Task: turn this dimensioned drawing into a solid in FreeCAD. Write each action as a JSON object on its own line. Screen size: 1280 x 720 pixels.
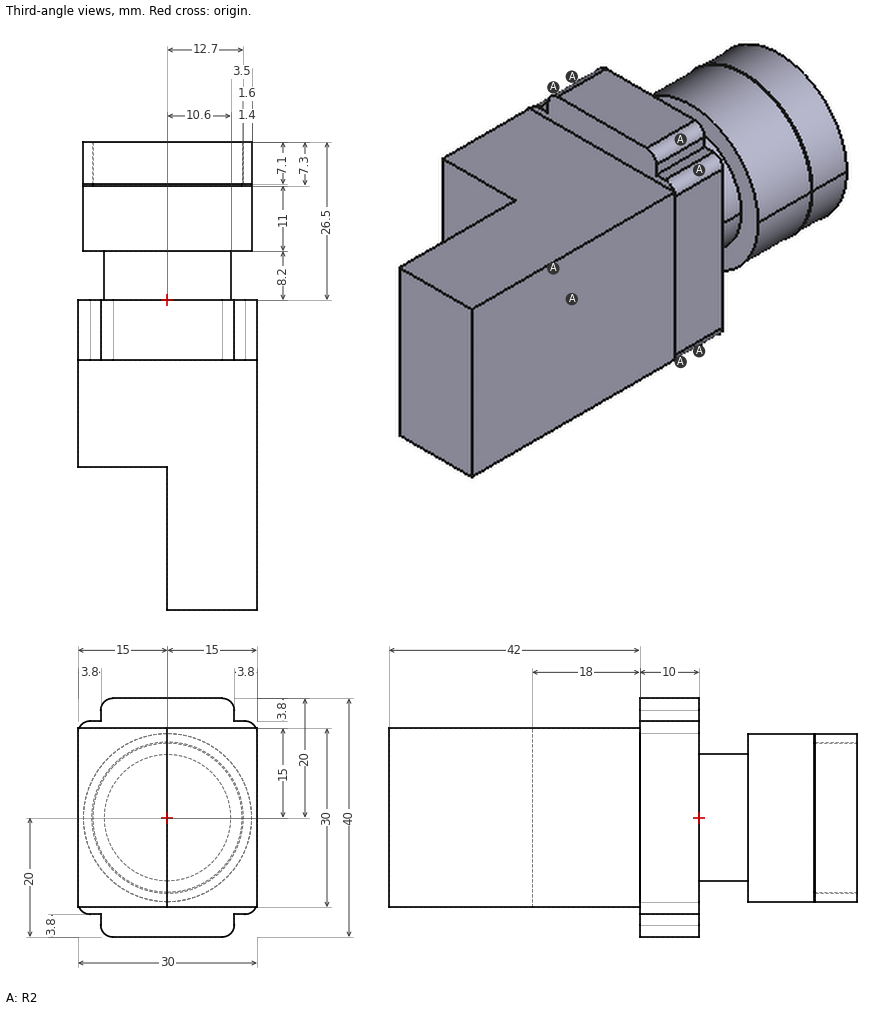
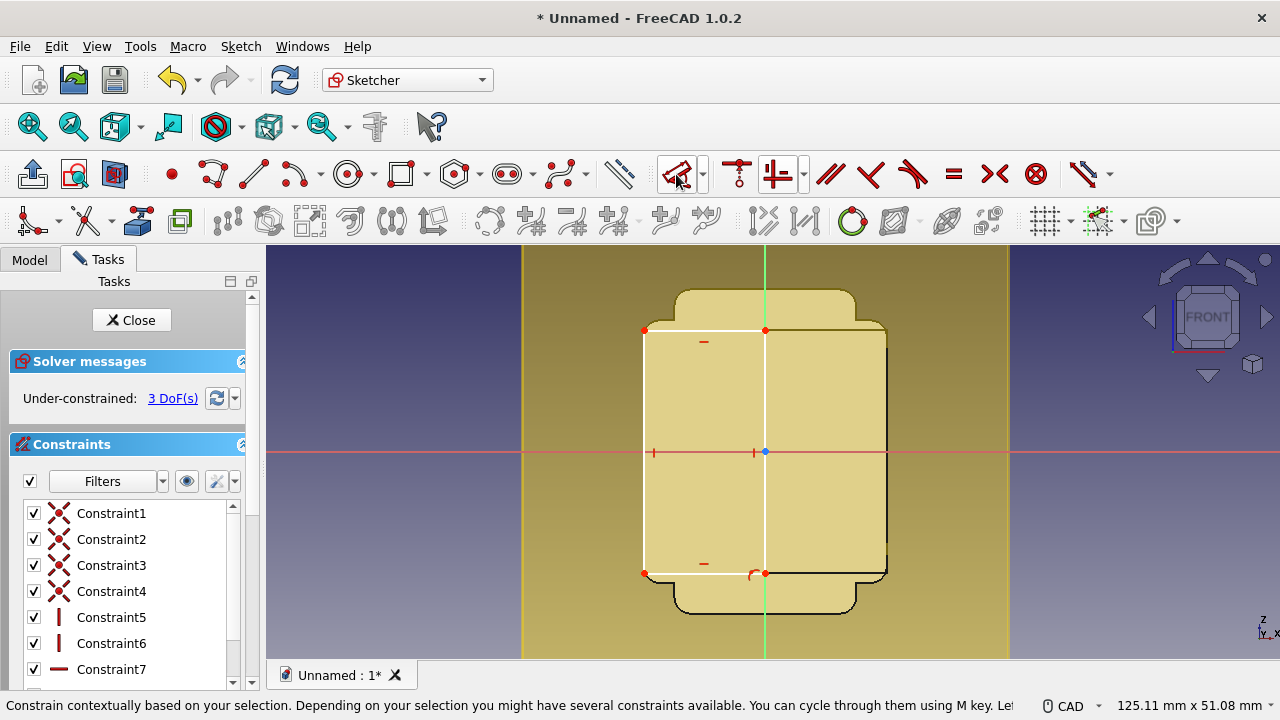
{"action": "left_click", "coordinate": [644, 404]}
{"action": "left_click", "coordinate": [610, 397]}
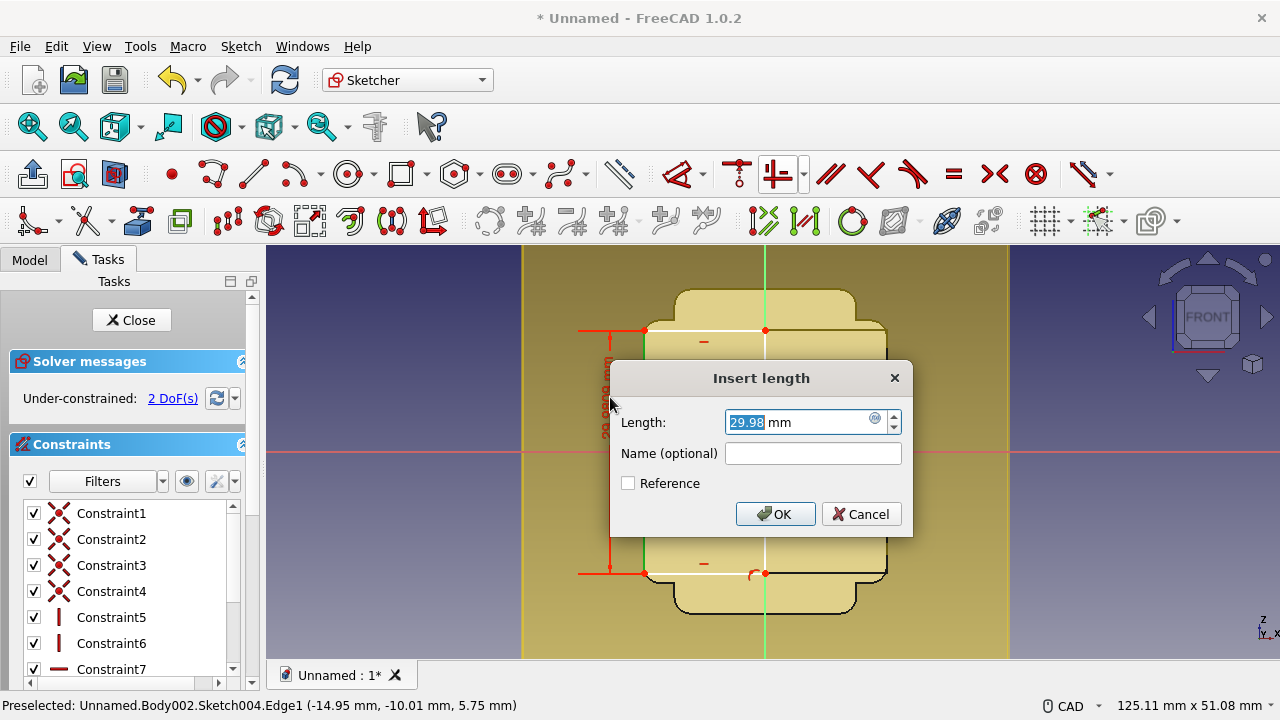
{"action": "type", "text": "30"}
{"action": "key", "text": "Return"}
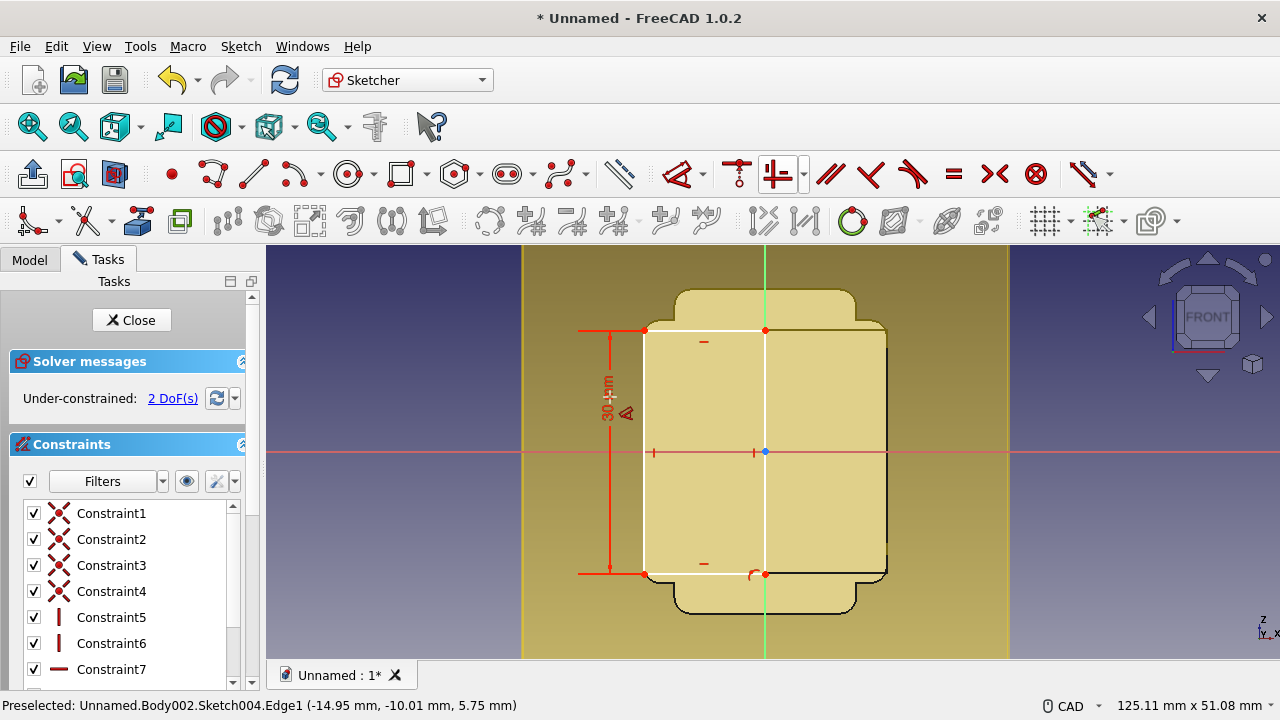
{"action": "left_click", "coordinate": [680, 574]}
{"action": "left_click", "coordinate": [705, 608]}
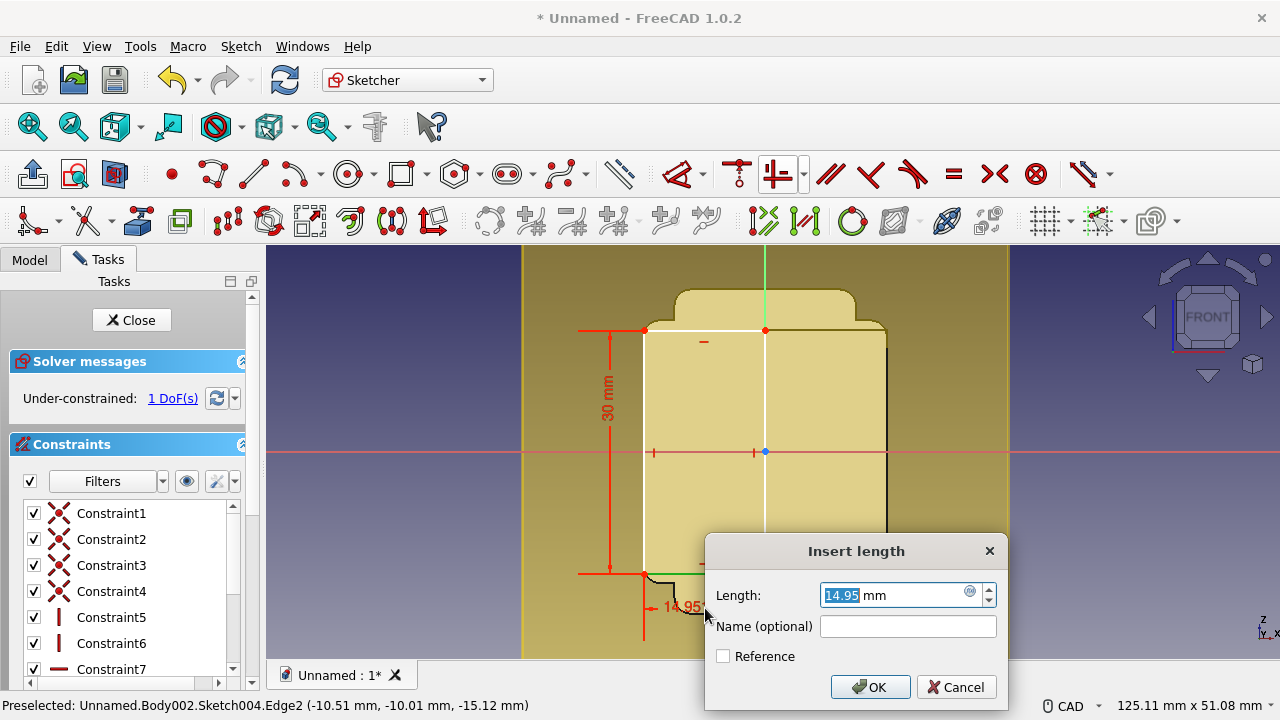
{"action": "type", "text": "15"}
{"action": "key", "text": "Return"}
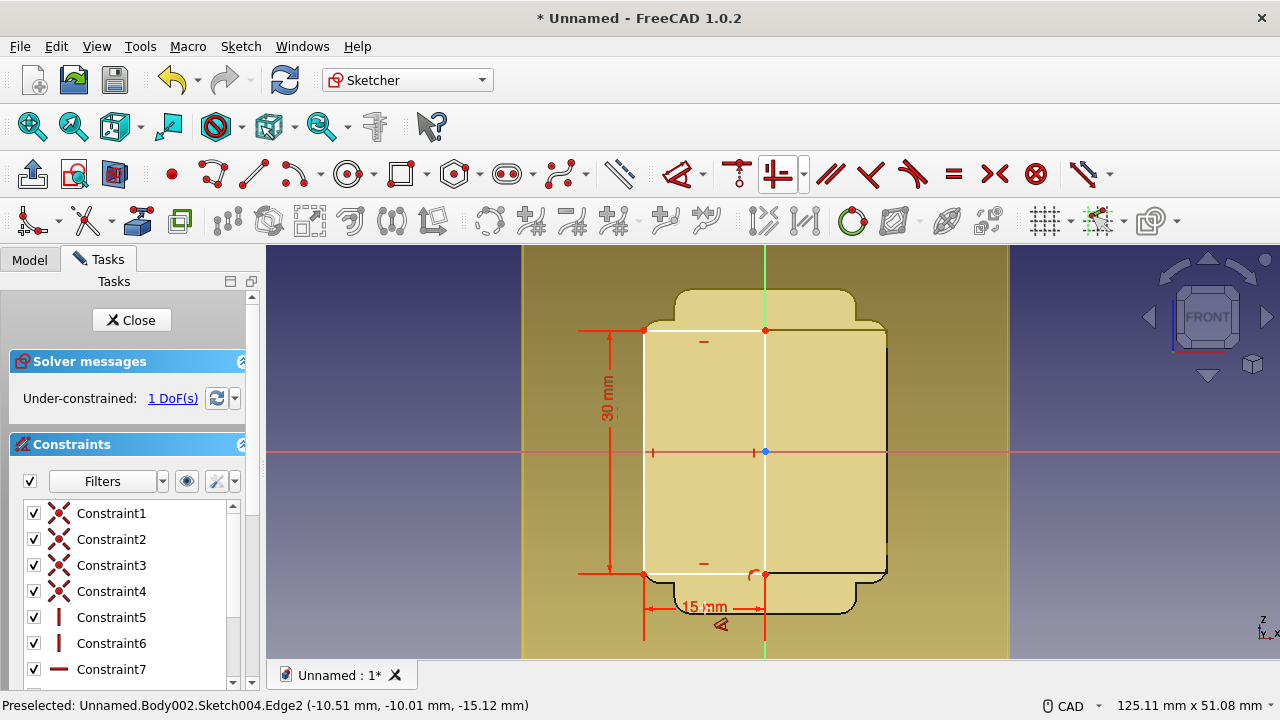
{"action": "left_click", "coordinate": [644, 331]}
{"action": "left_click", "coordinate": [799, 391]}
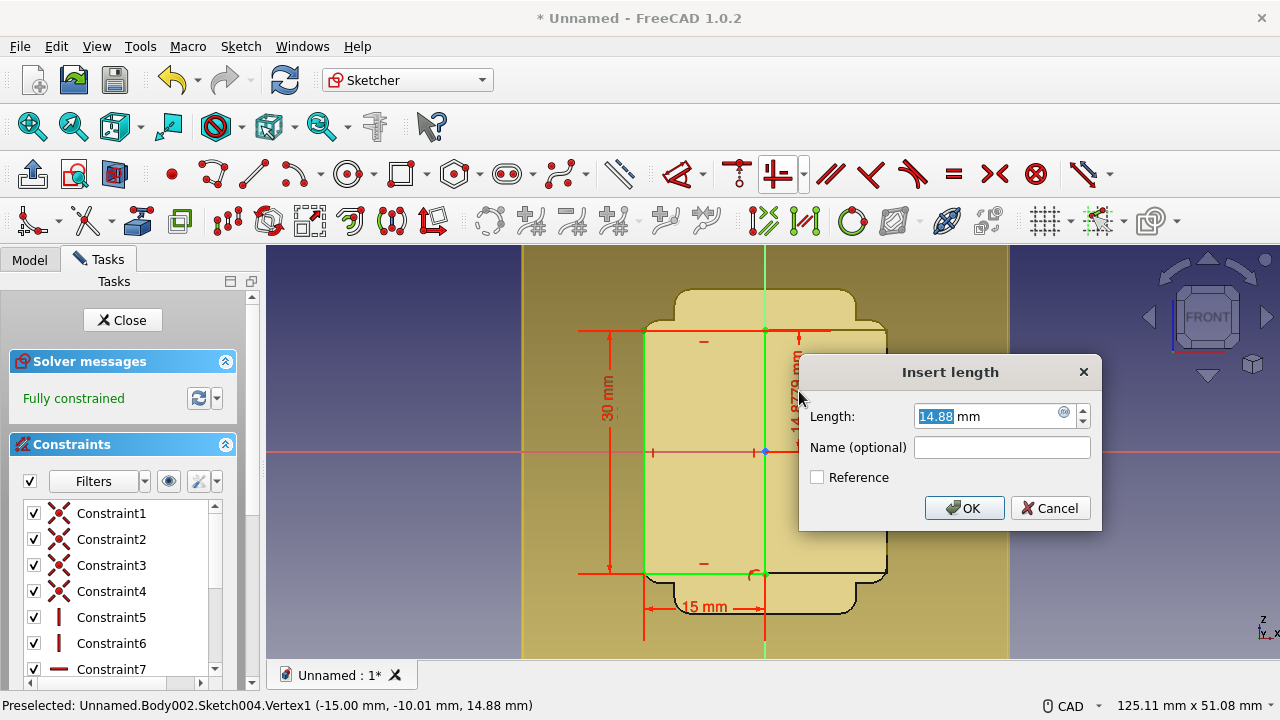
{"action": "type", "text": "15"}
{"action": "key", "text": "Return"}
{"action": "key", "text": "Escape"}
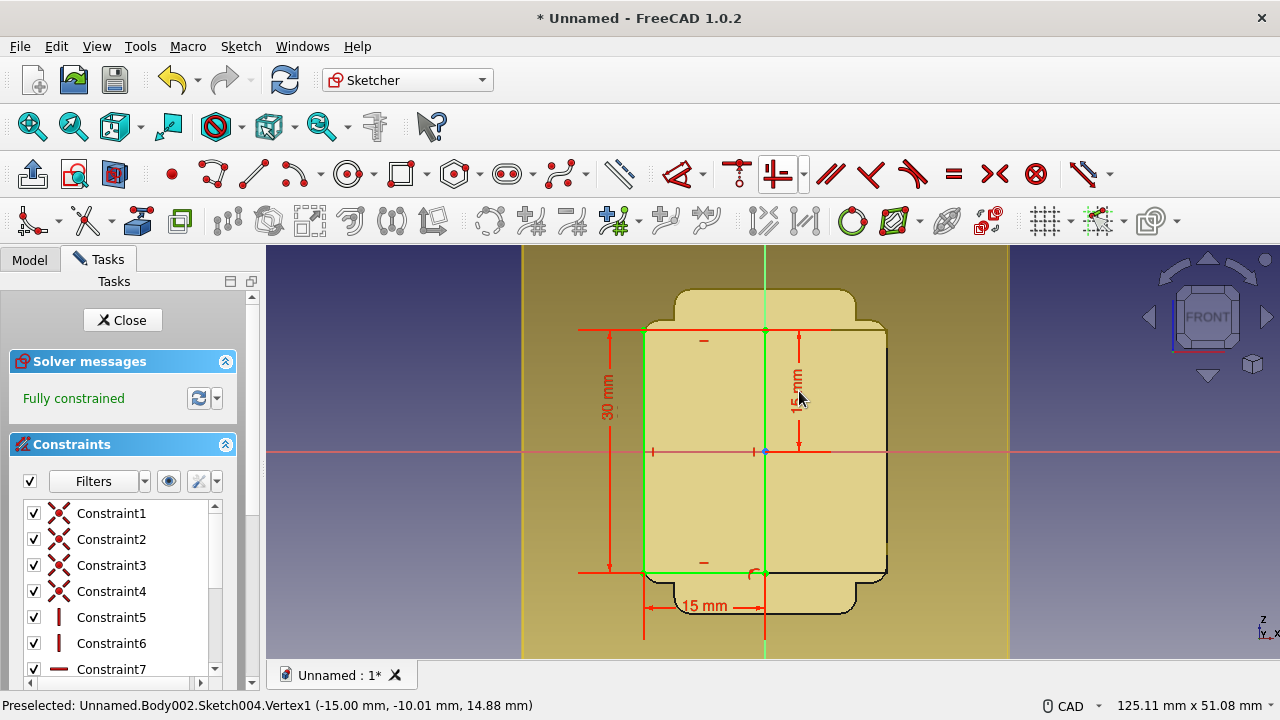
{"action": "left_click", "coordinate": [123, 320]}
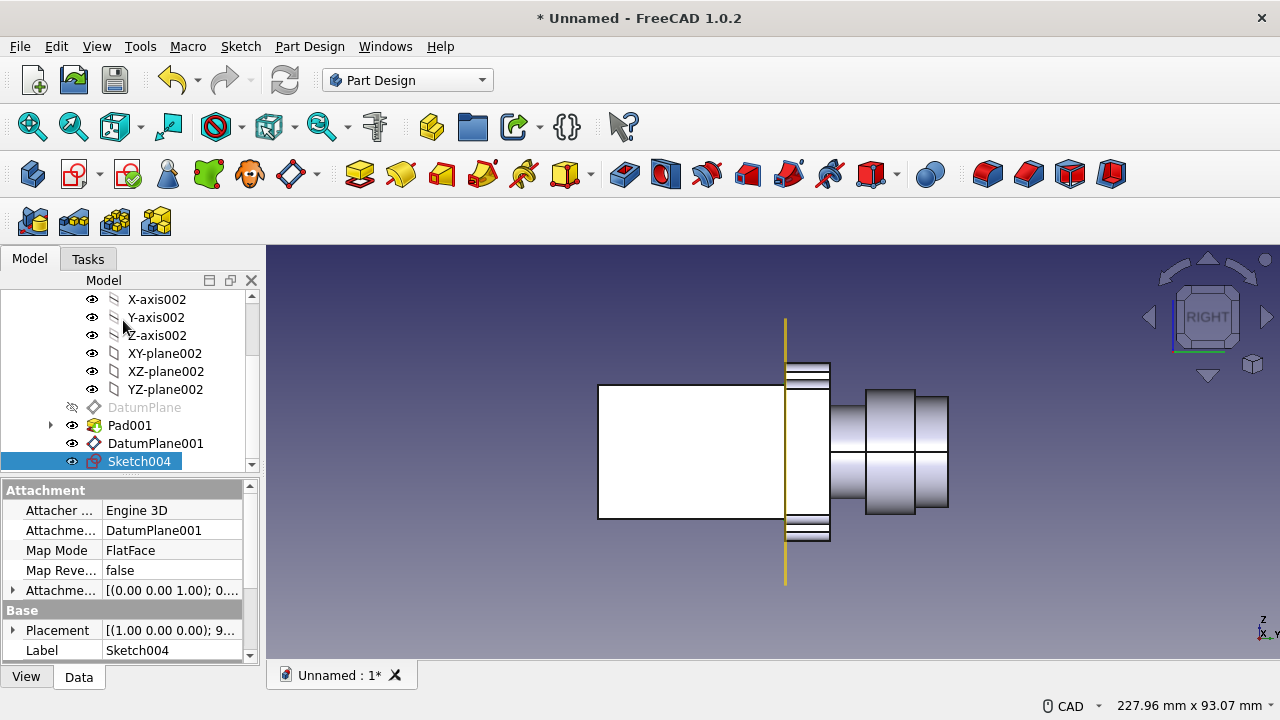
{"action": "left_click", "coordinate": [360, 174]}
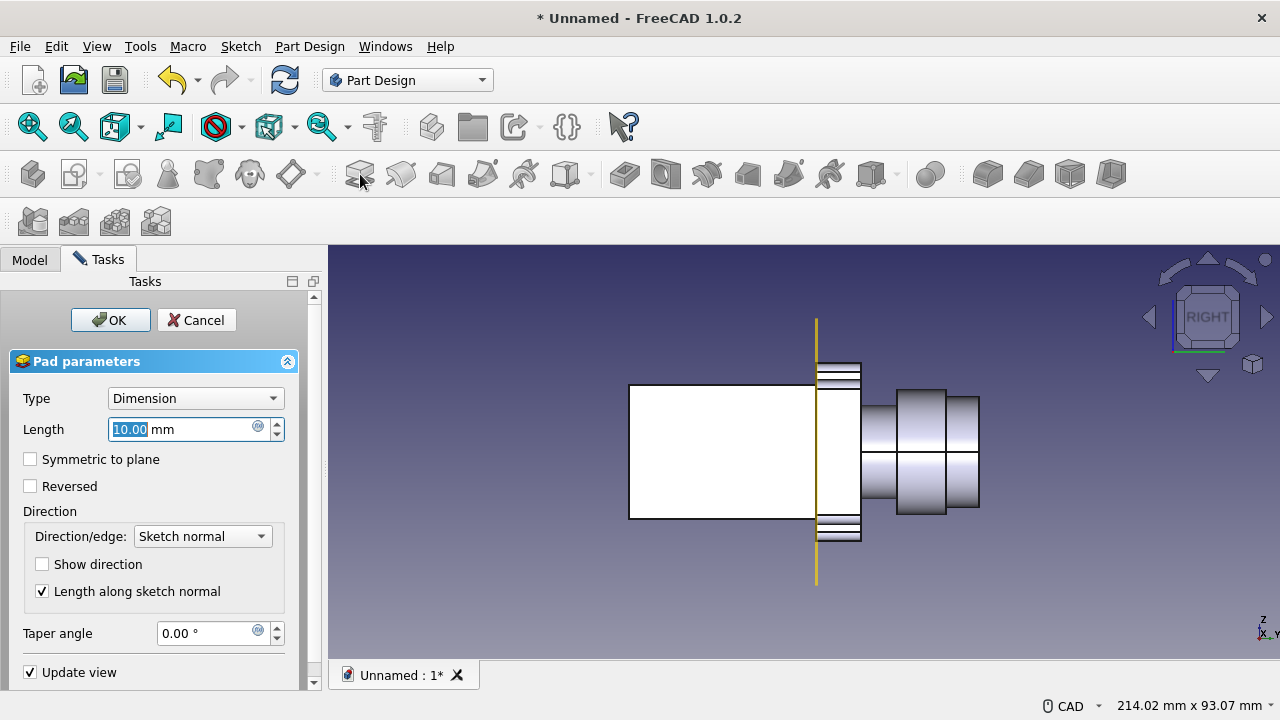
{"action": "type", "text": "18"}
{"action": "key", "text": "Tab"}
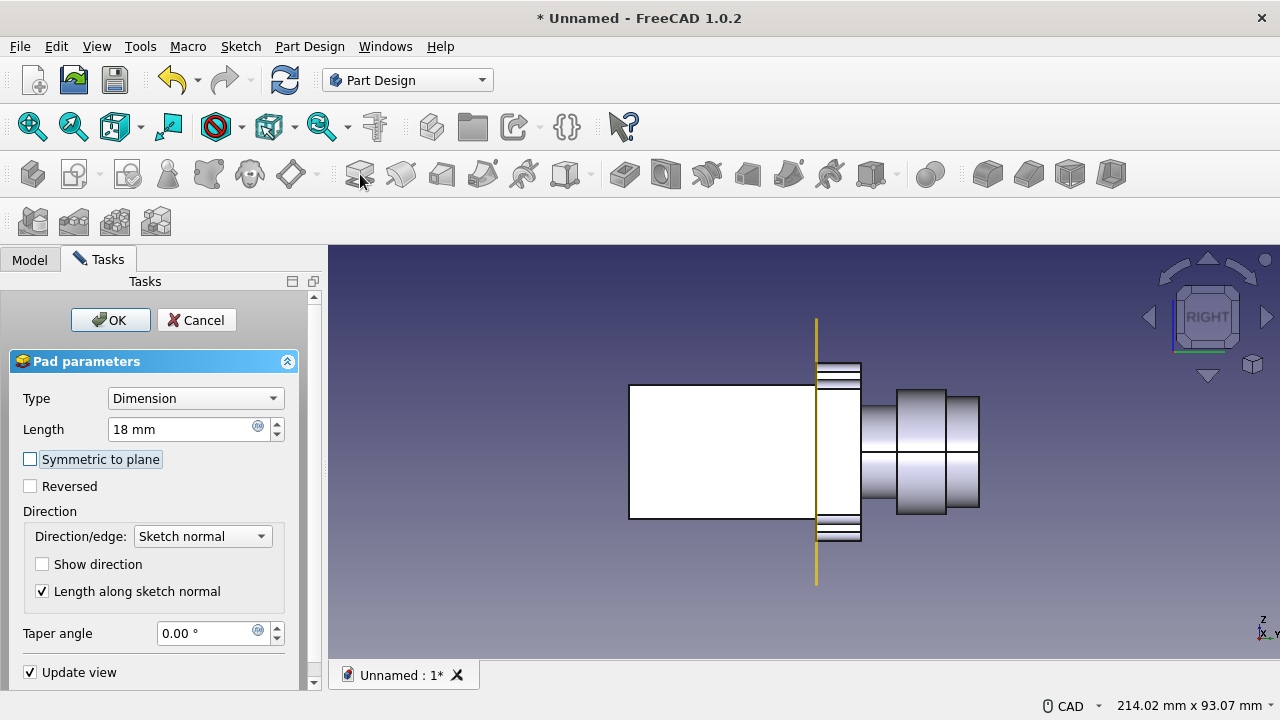
{"action": "left_click", "coordinate": [111, 320]}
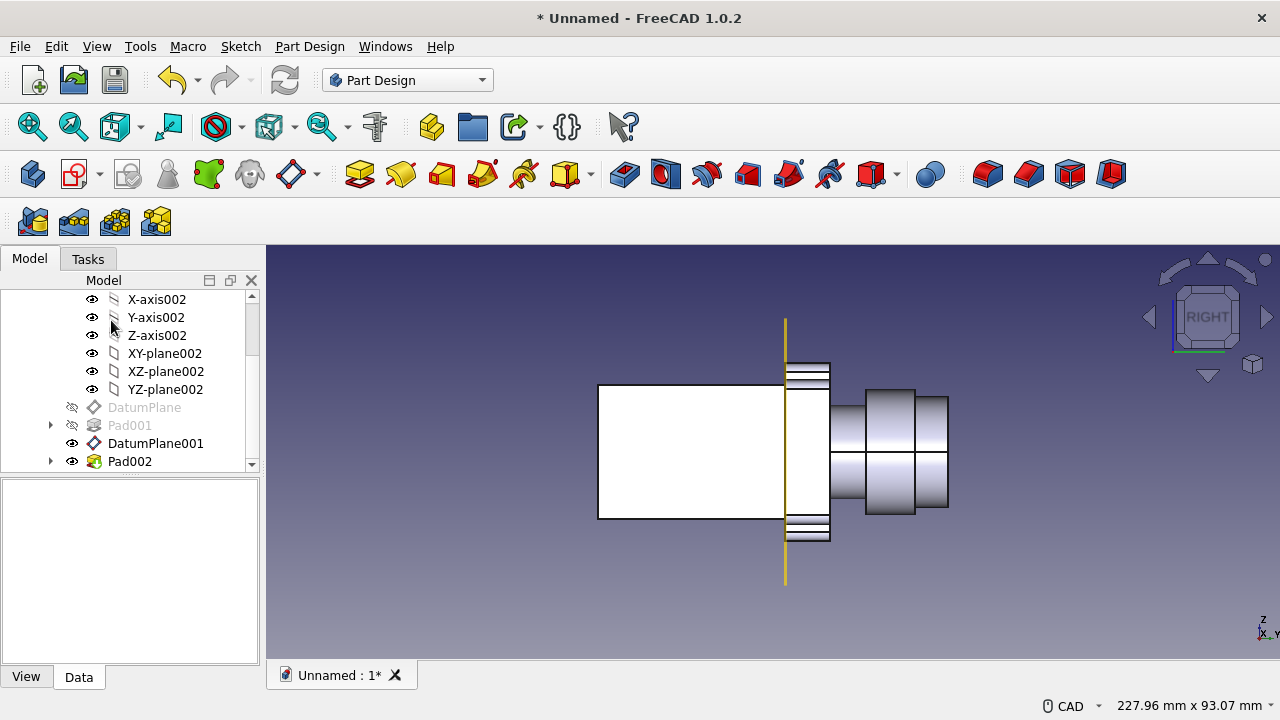
{"action": "left_click", "coordinate": [117, 443]}
{"action": "key", "text": "space"}